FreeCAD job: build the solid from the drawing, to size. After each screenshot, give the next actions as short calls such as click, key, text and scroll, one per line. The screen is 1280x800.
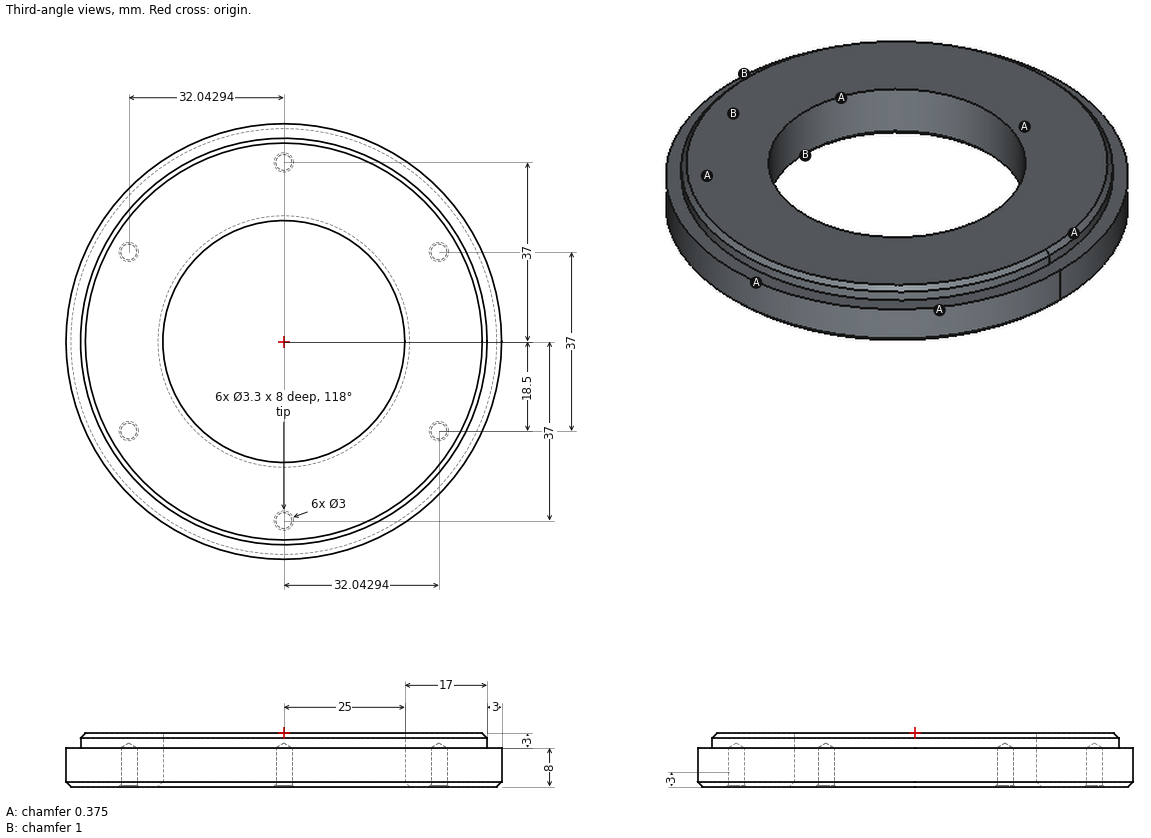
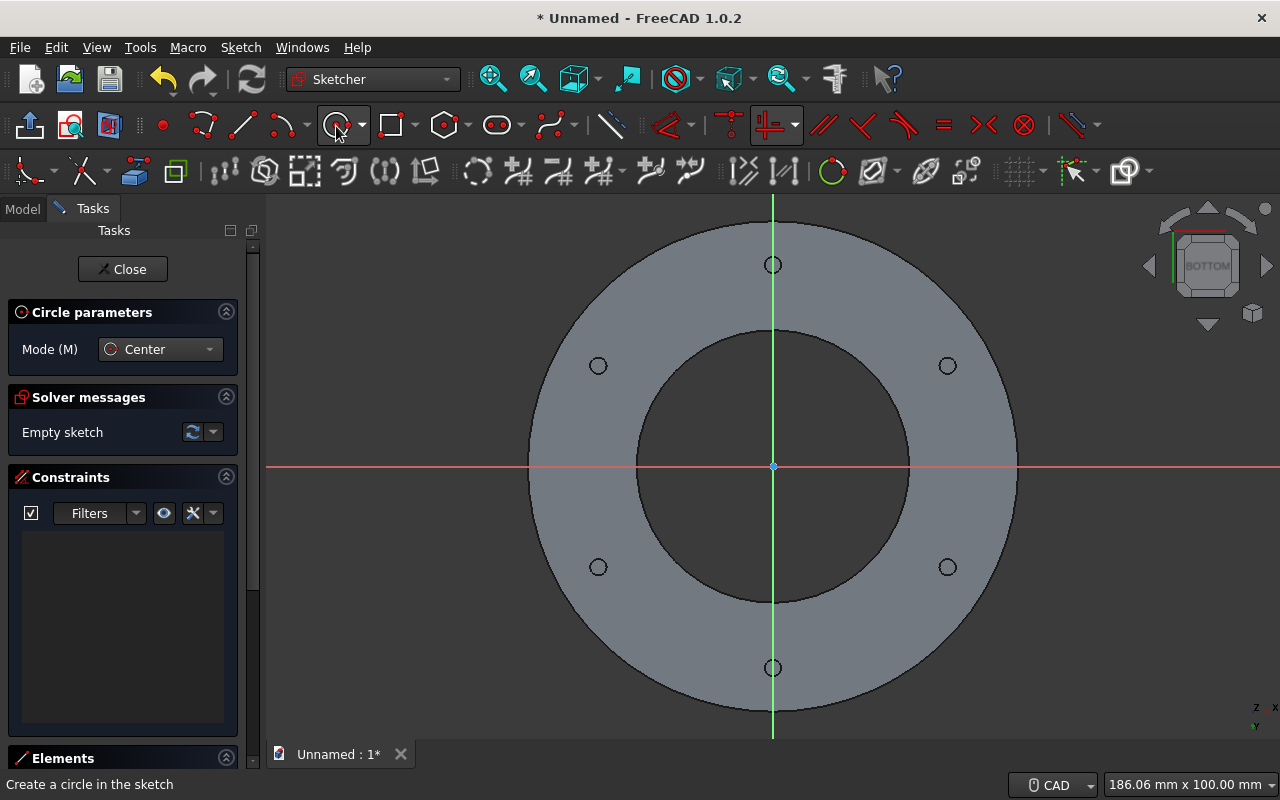
scroll(773, 265, up, 5)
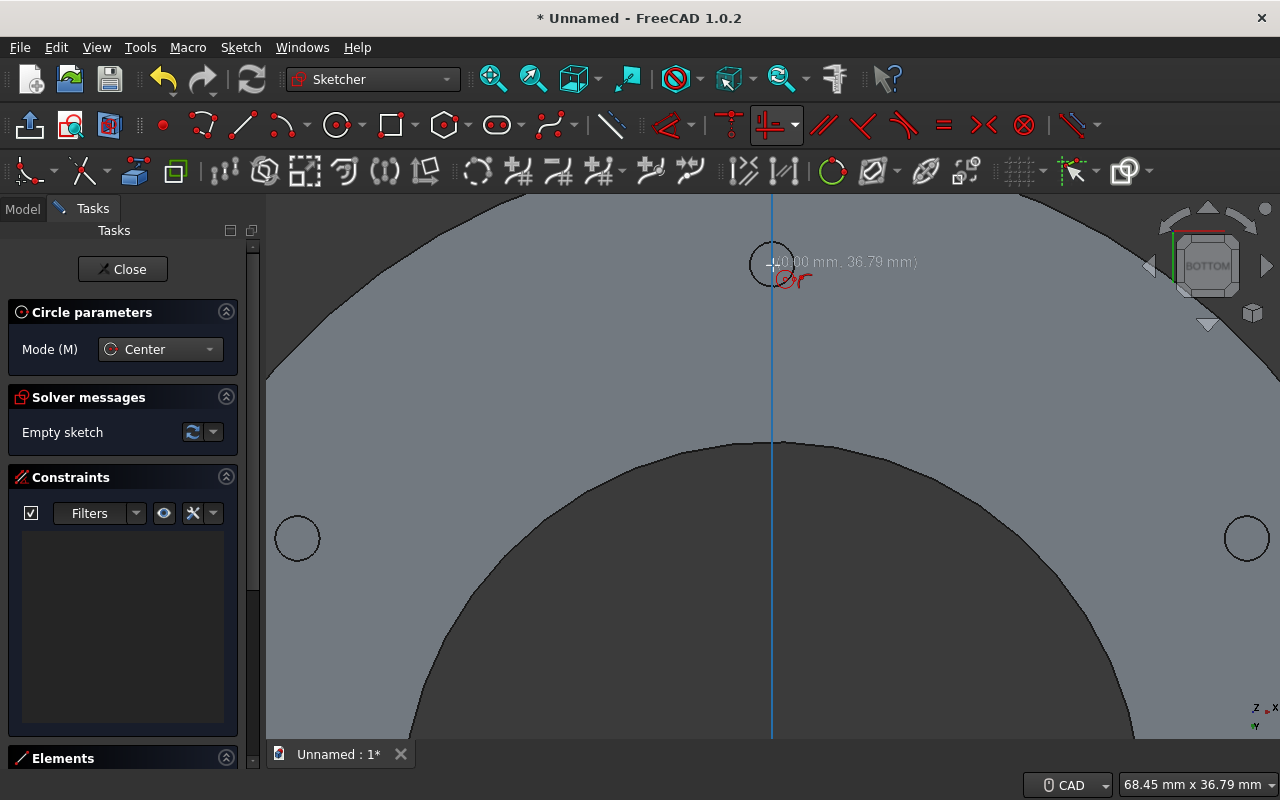
click(772, 264)
move(789, 247)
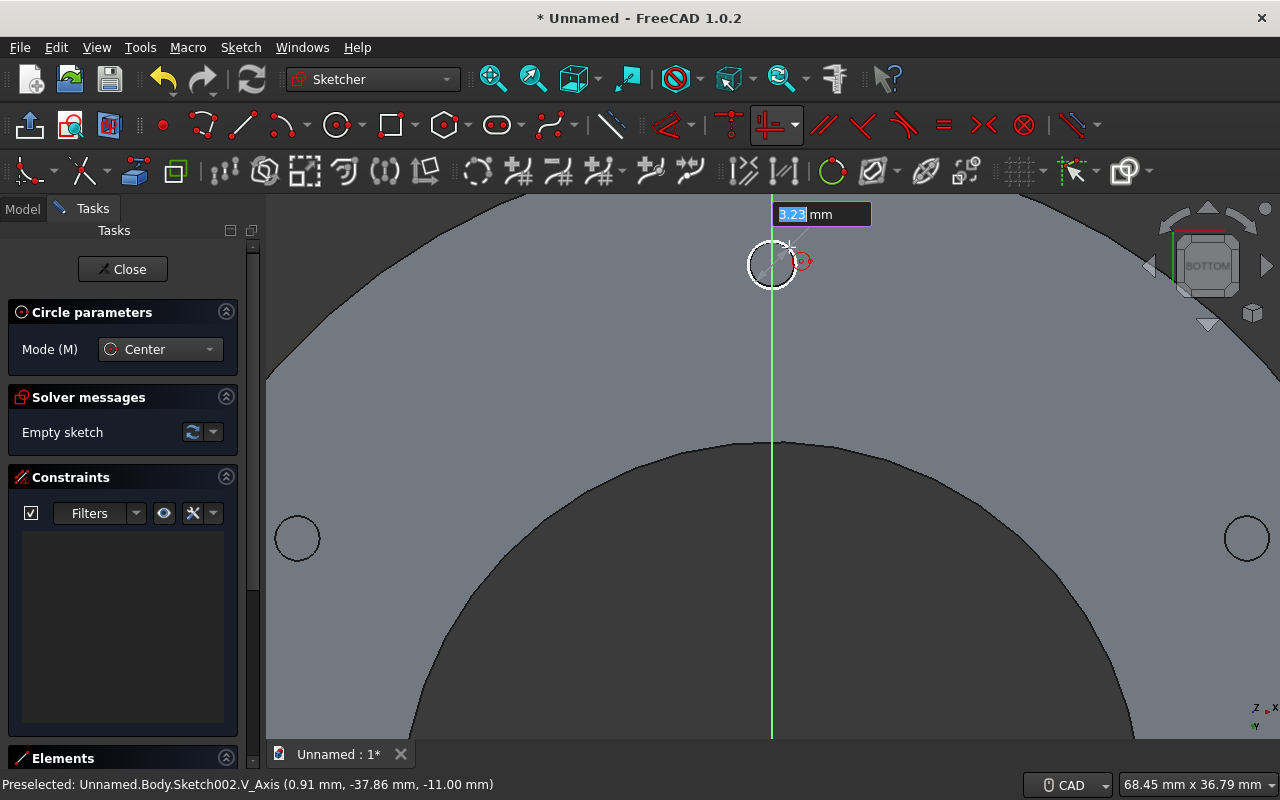
text(3.3)
key(Return)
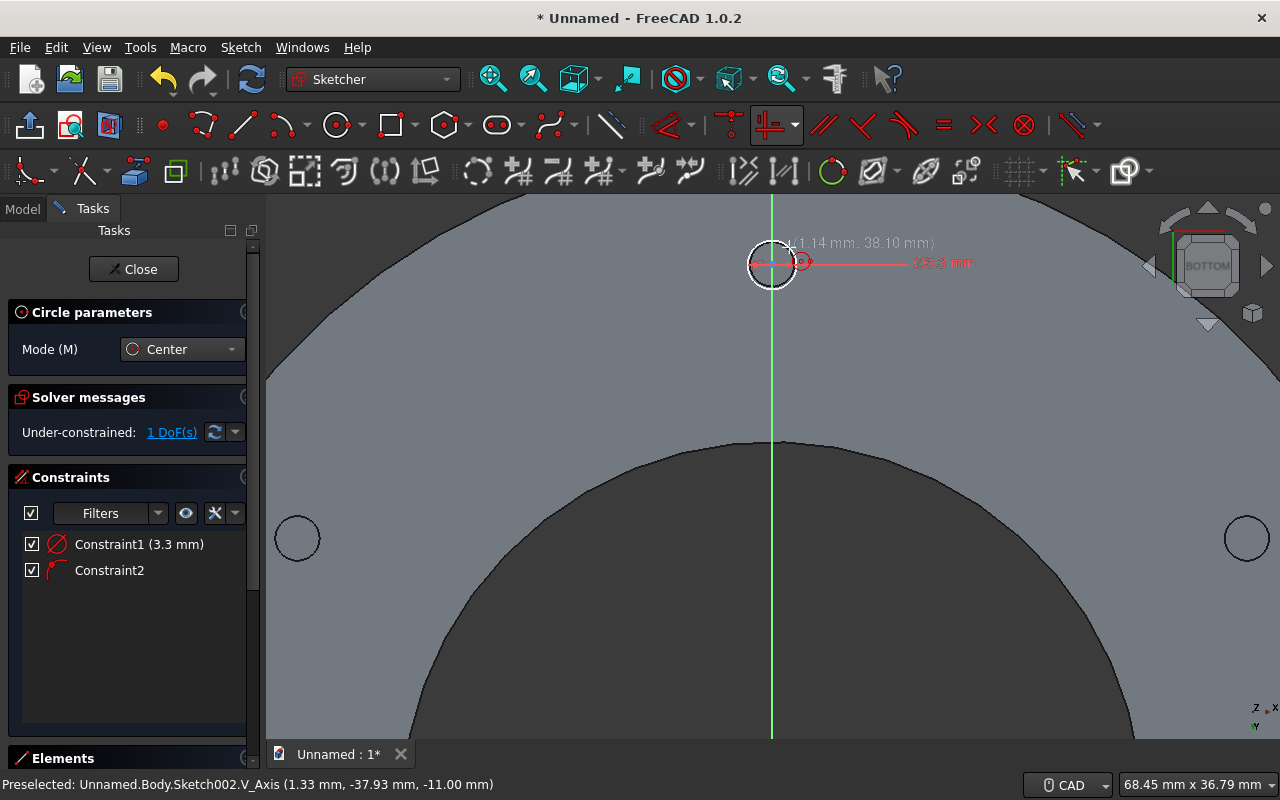
scroll(675, 317, down, 6)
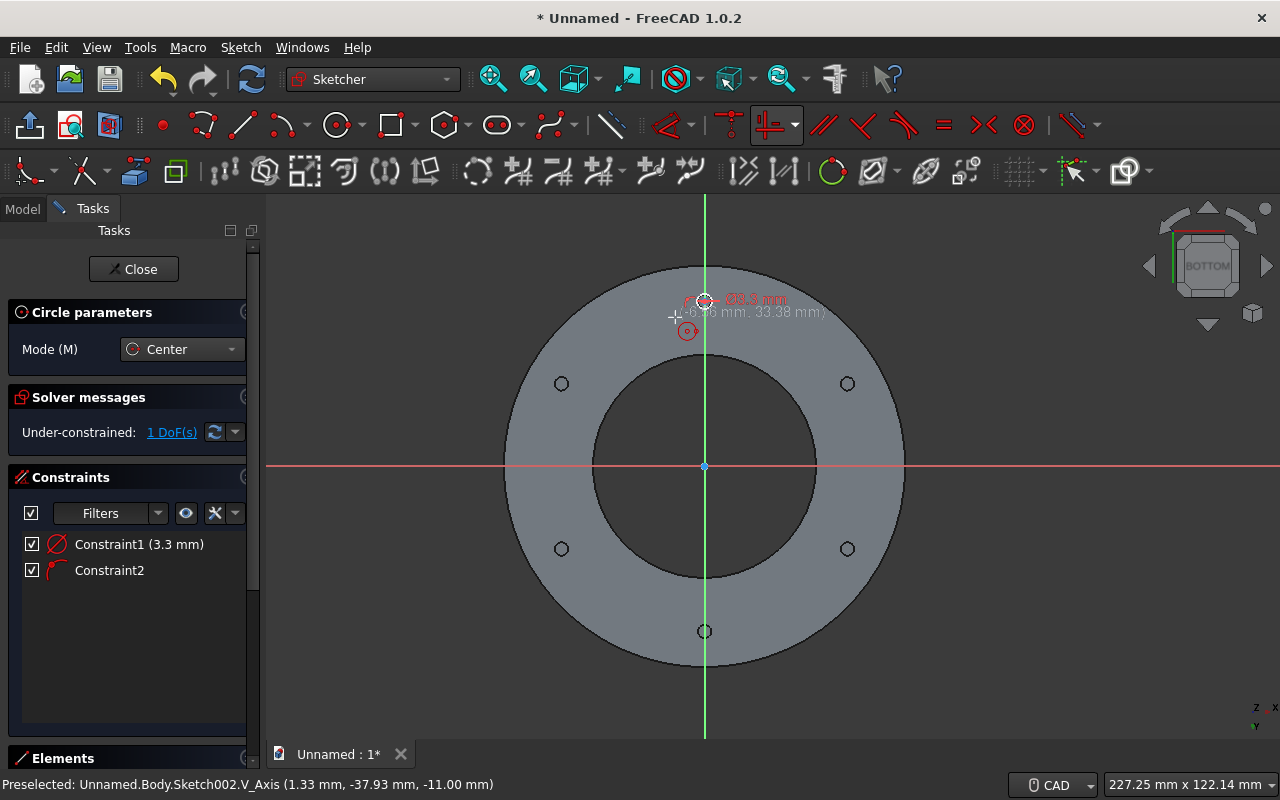
scroll(848, 384, up, 6)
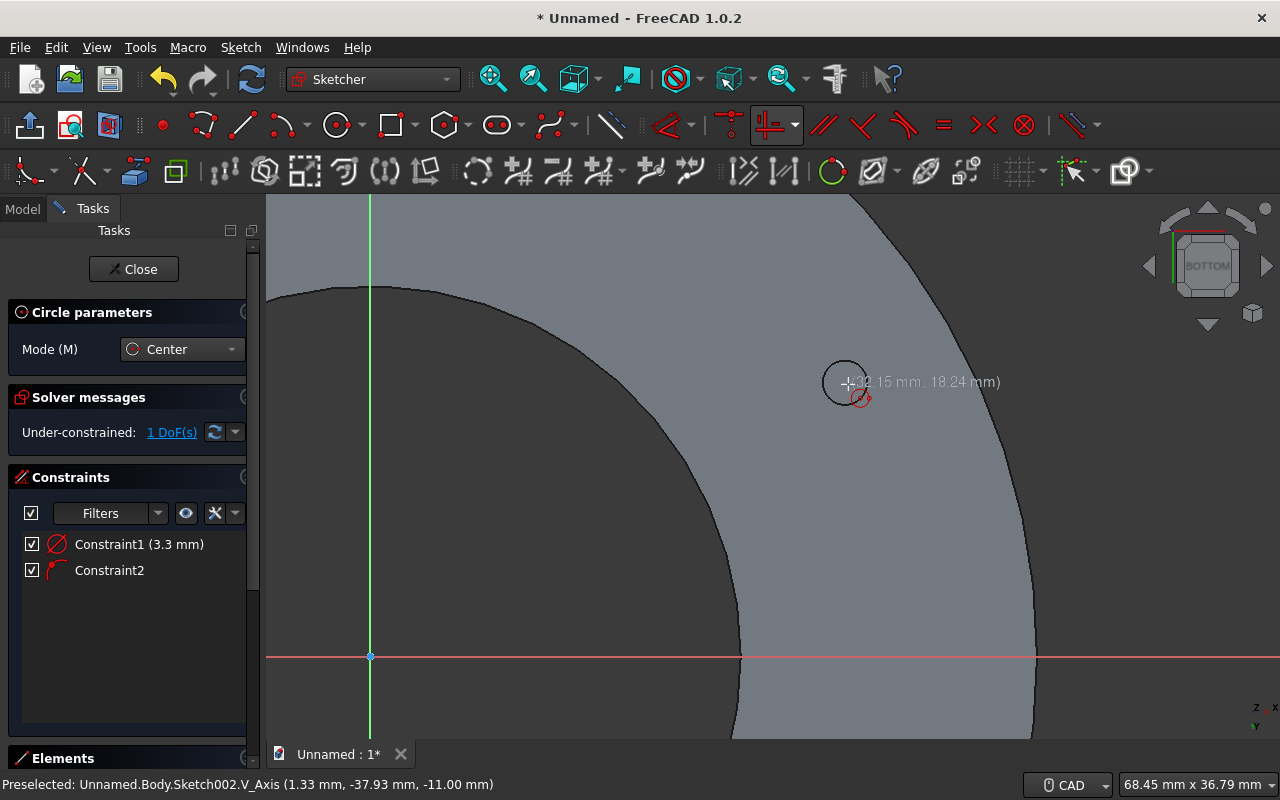
click(845, 383)
move(862, 365)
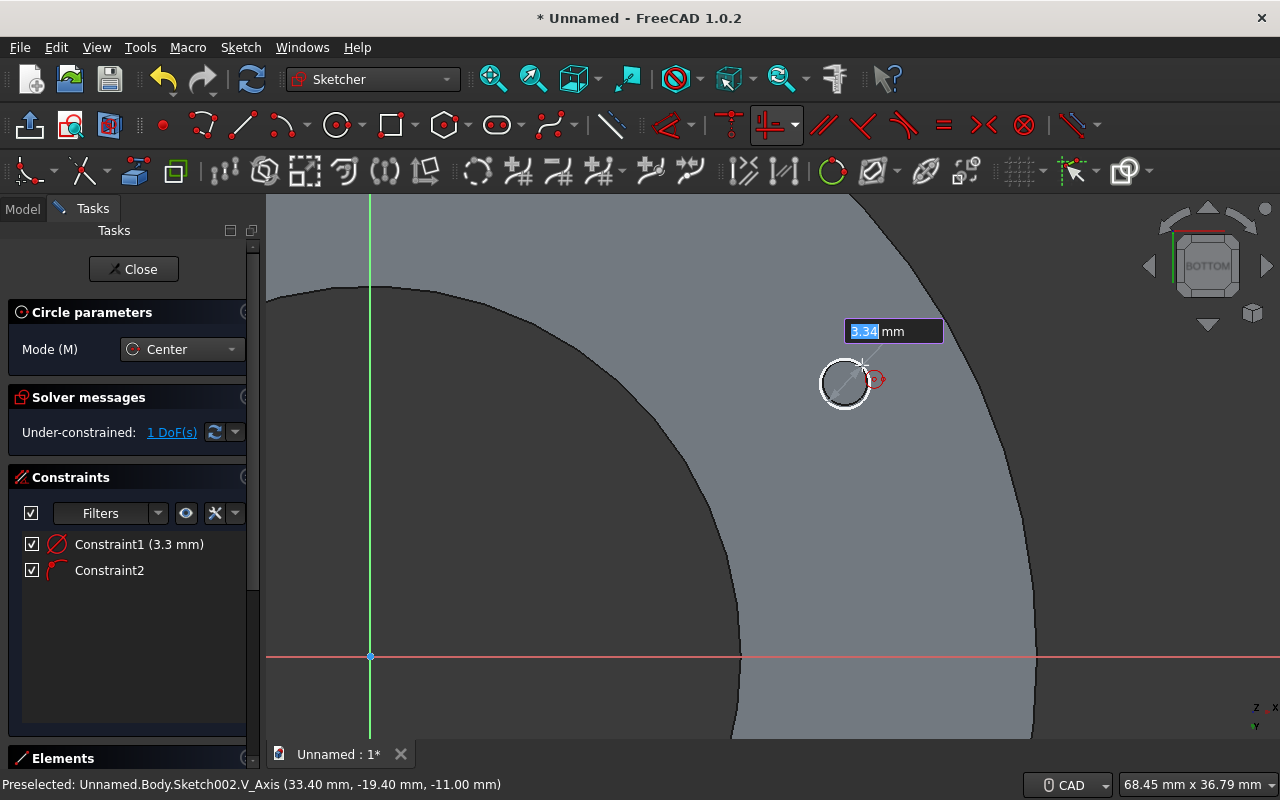
text(3.3)
key(Return)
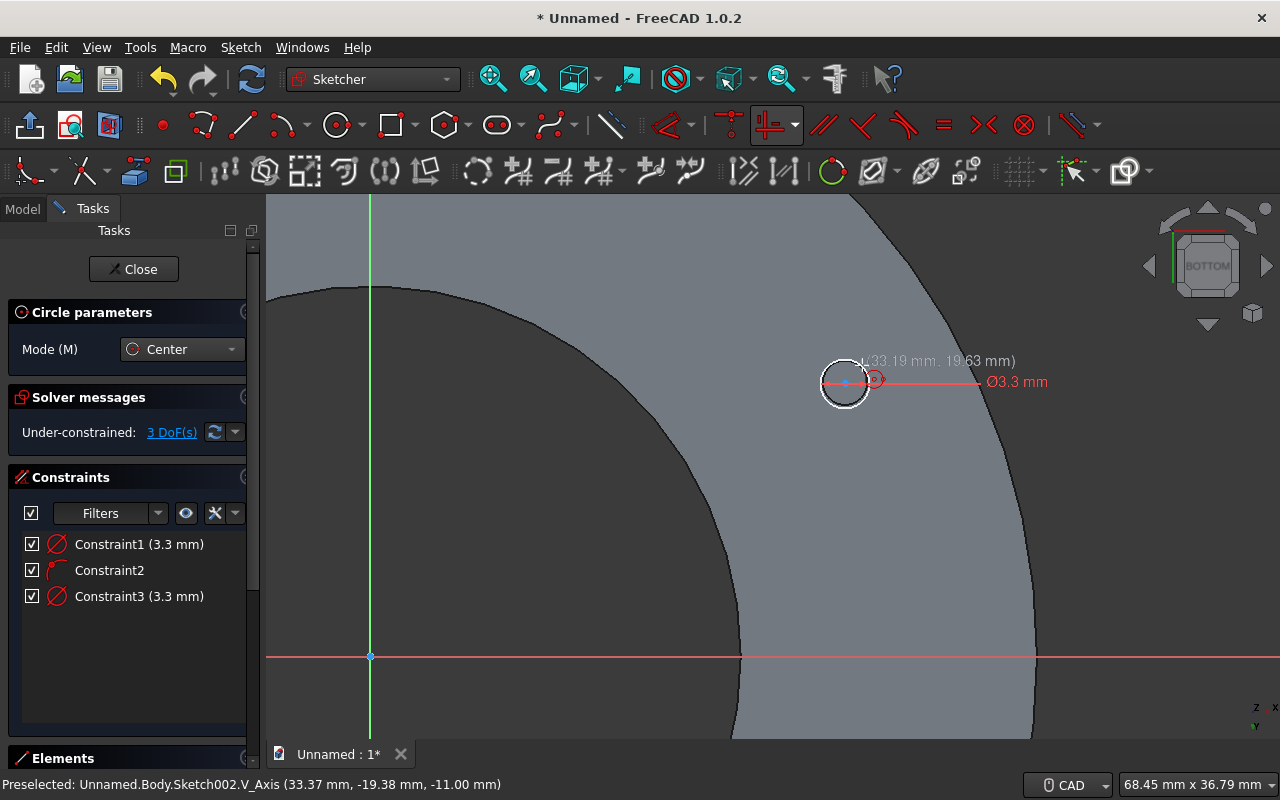
scroll(849, 384, down, 6)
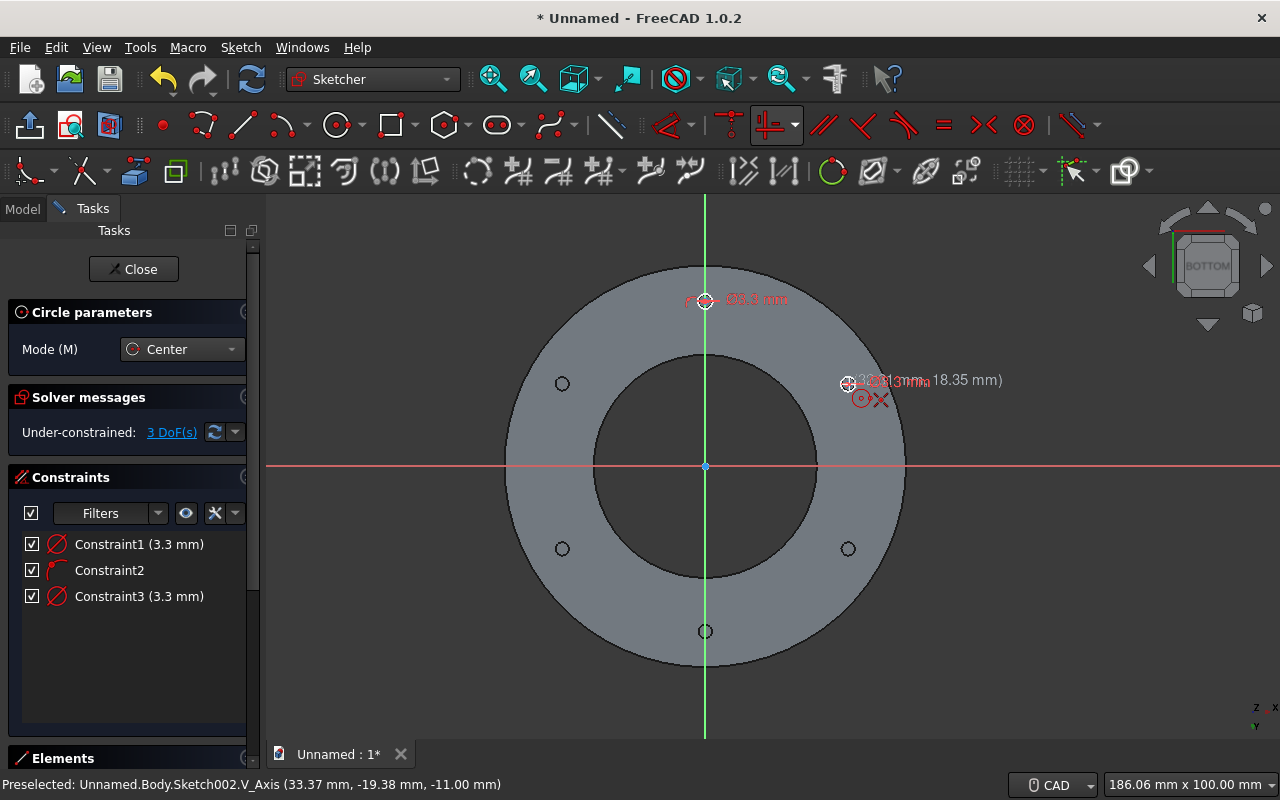
scroll(848, 549, up, 6)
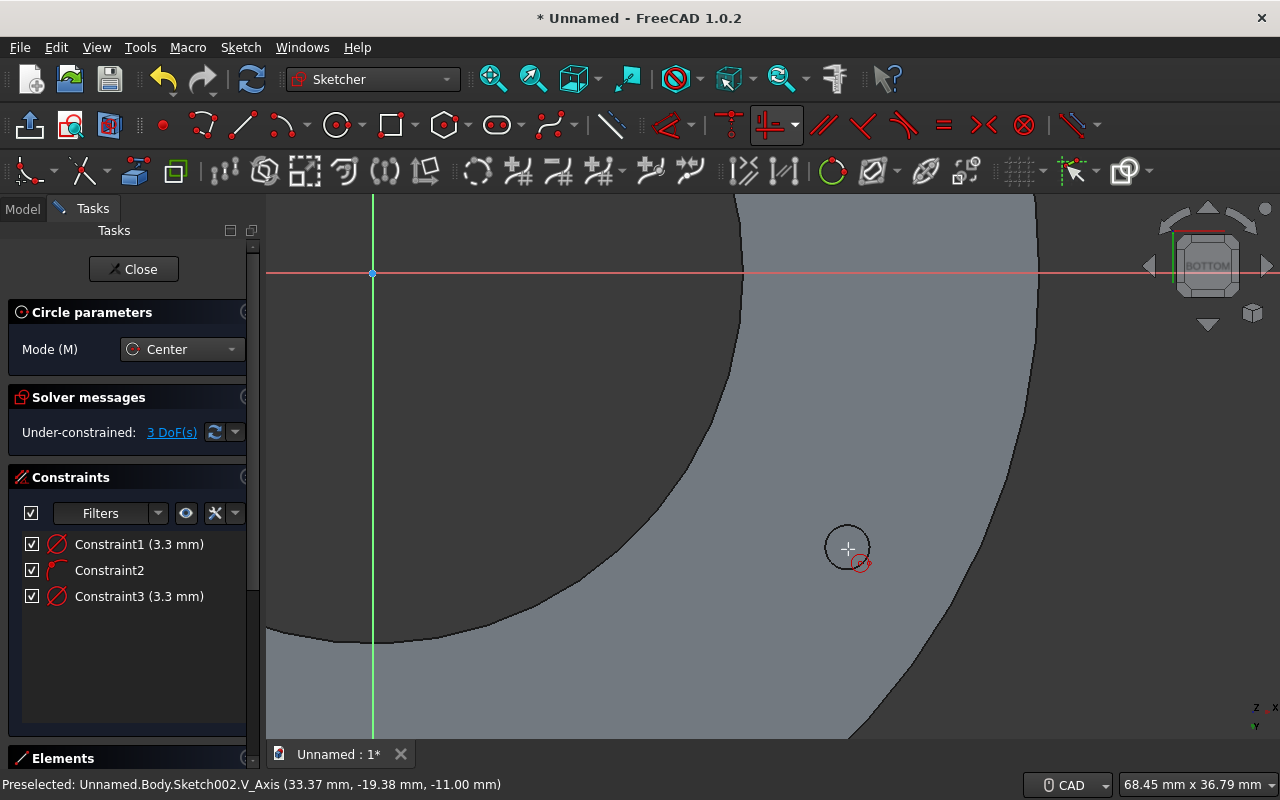
click(847, 547)
move(865, 530)